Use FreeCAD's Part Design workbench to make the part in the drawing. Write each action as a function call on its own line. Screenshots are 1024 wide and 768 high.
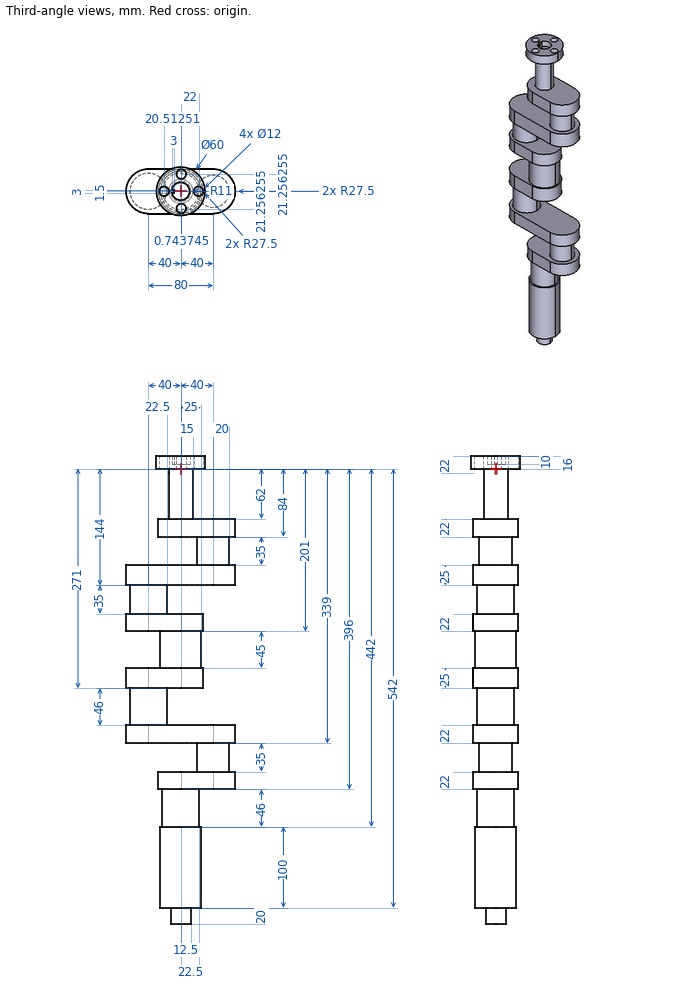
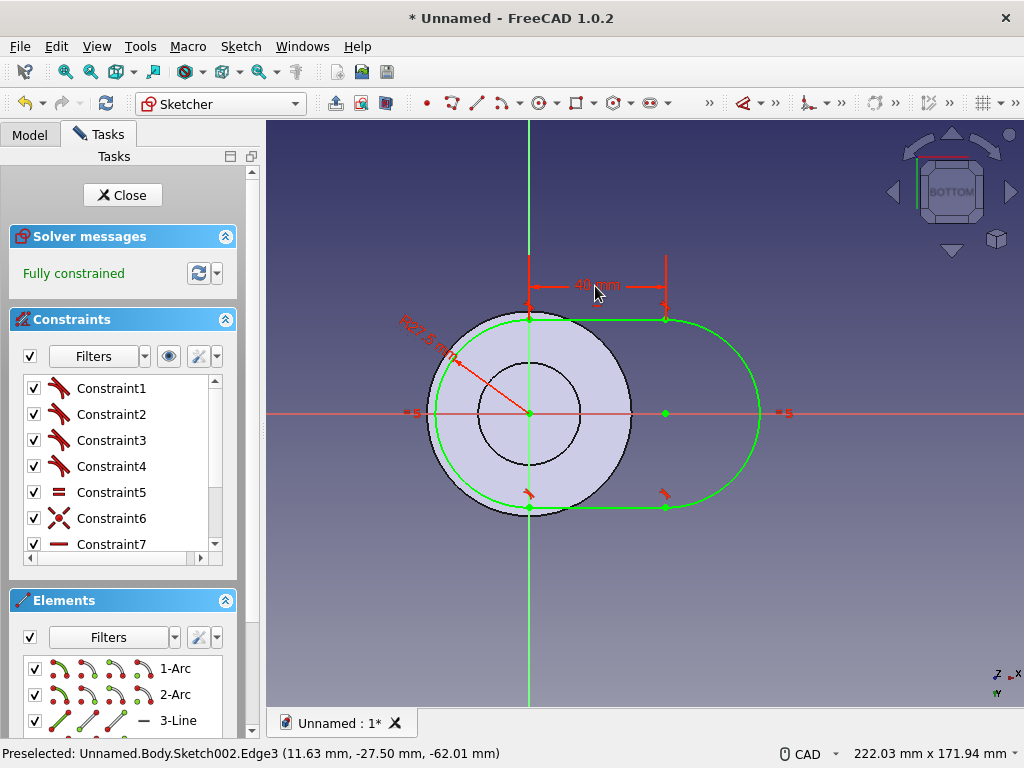
click(123, 195)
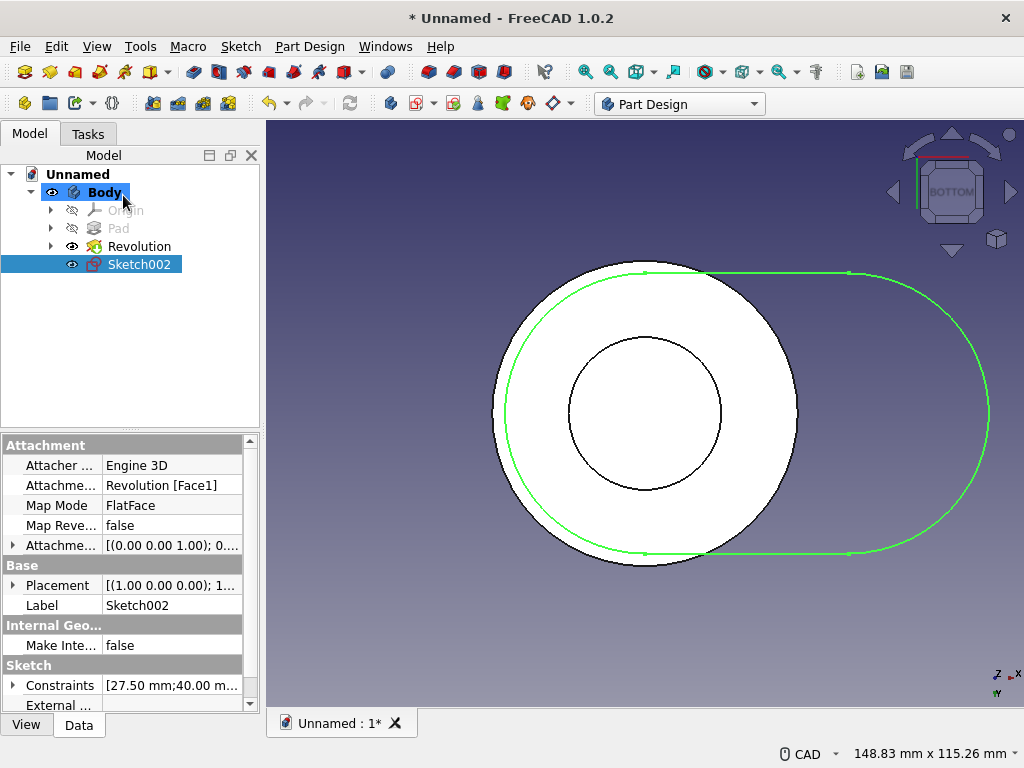
click(25, 72)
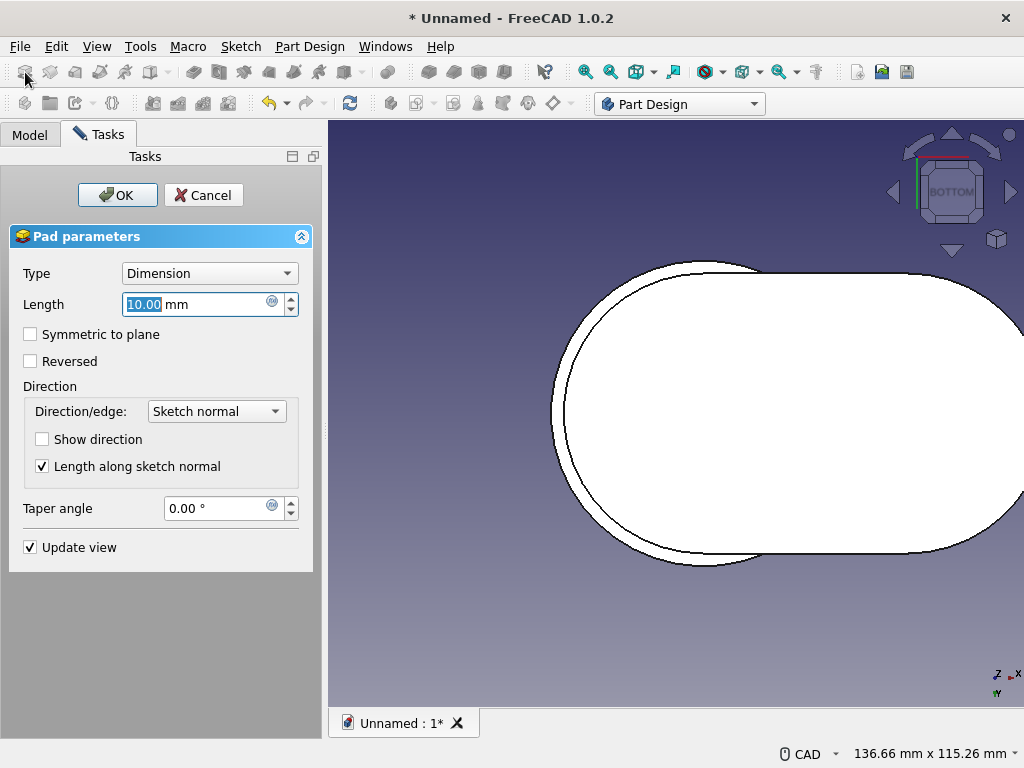
text(22)
key(Tab)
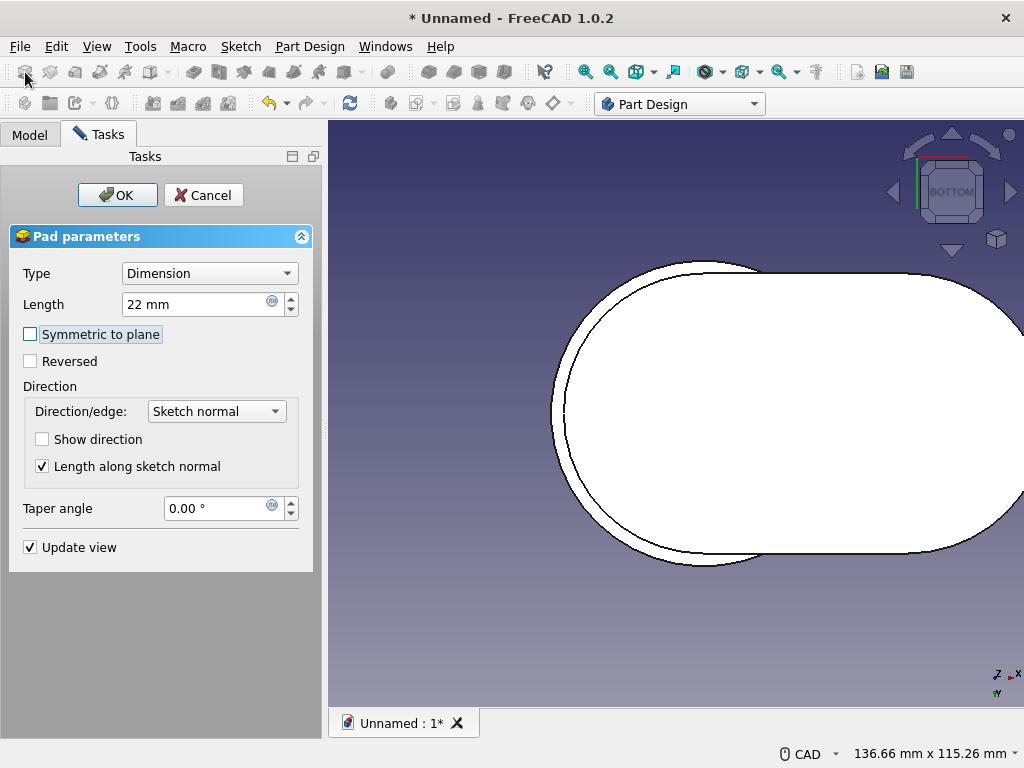
click(118, 195)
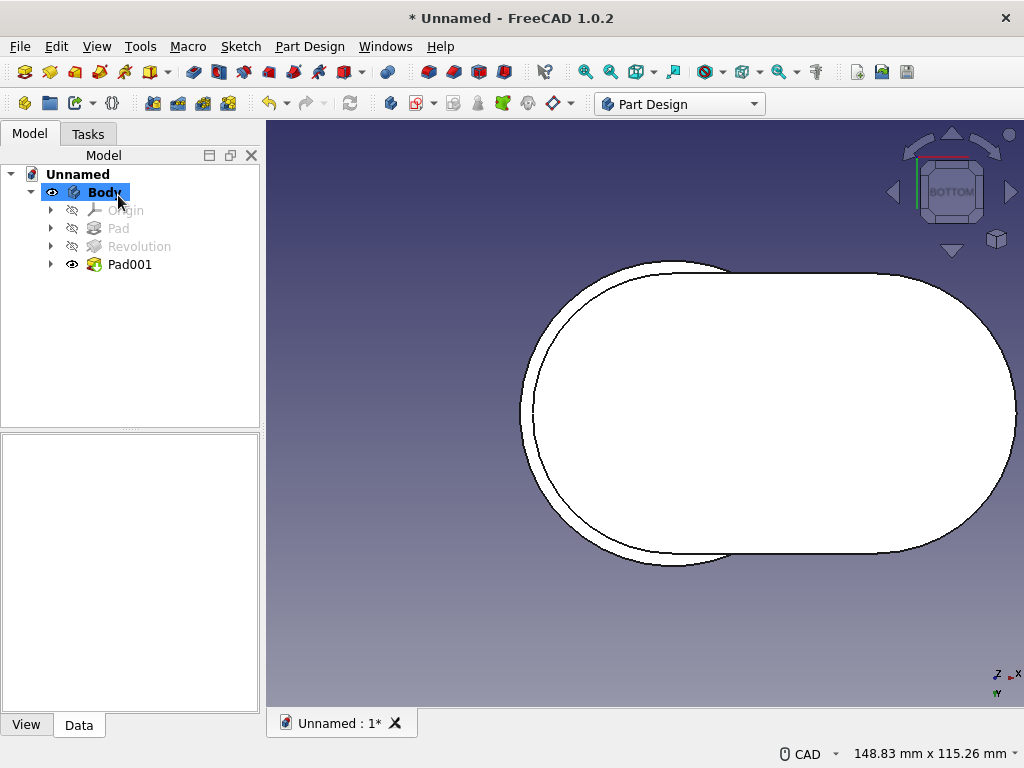
click(416, 104)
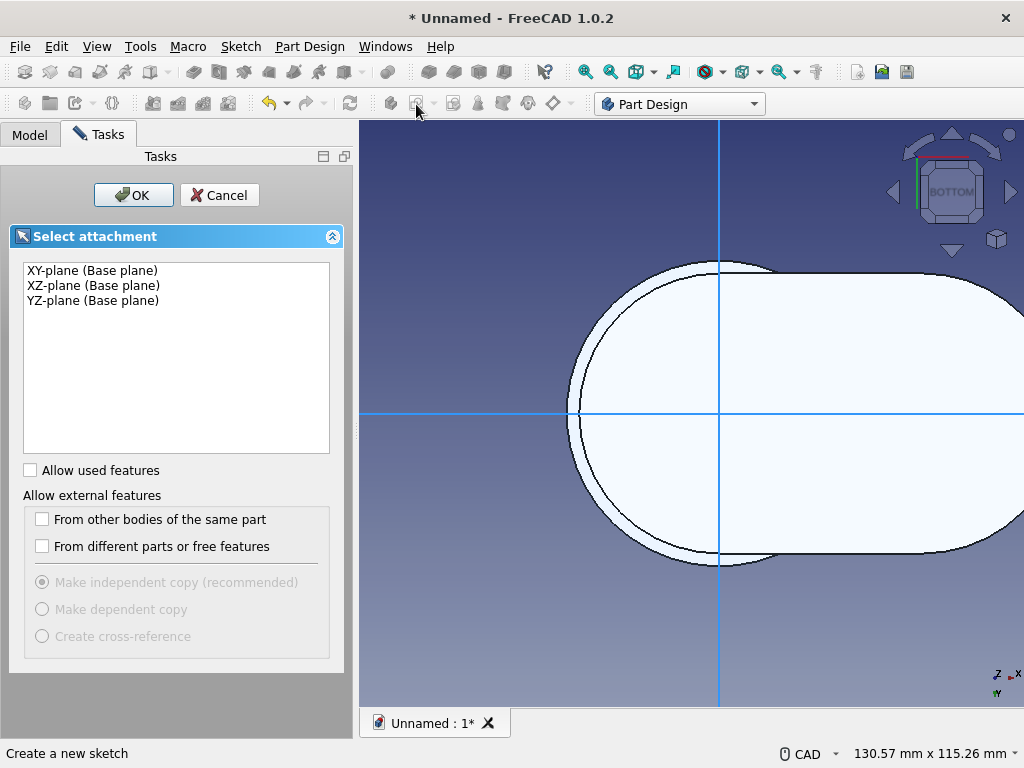
click(84, 286)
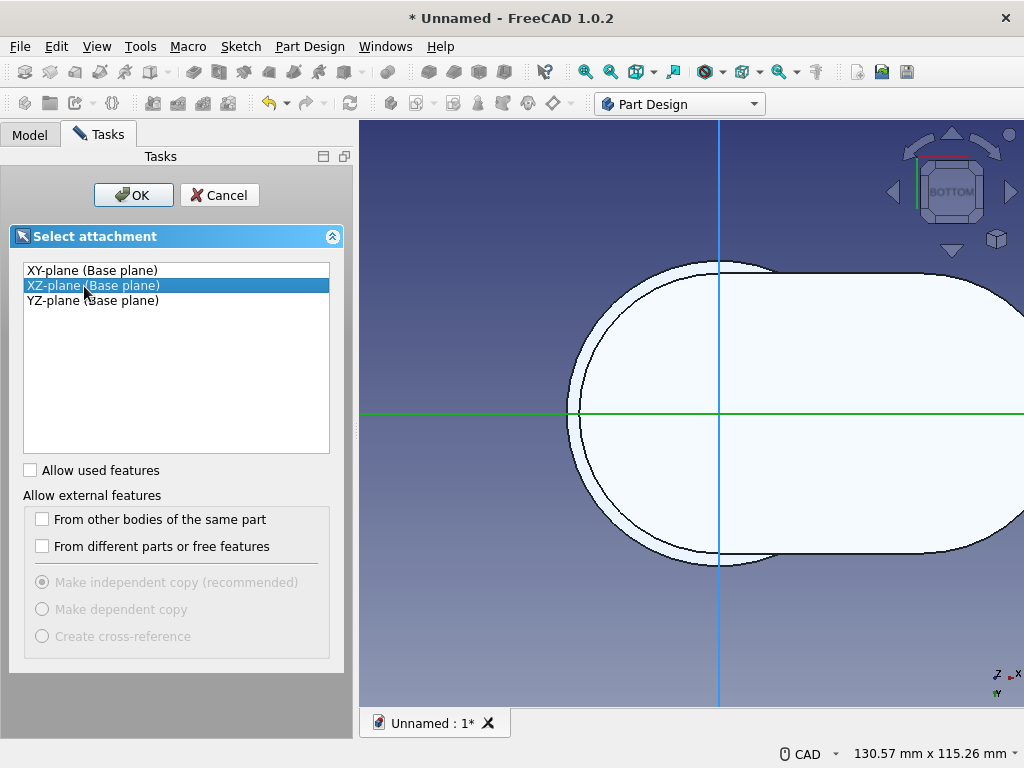
click(134, 195)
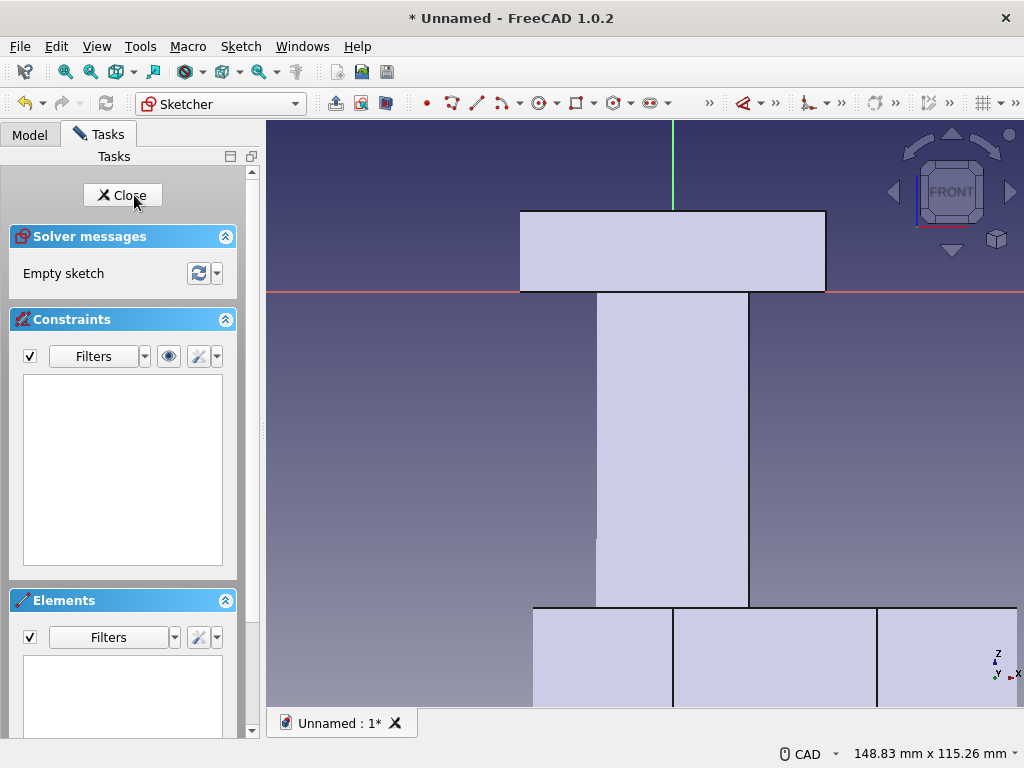
key(q)
key(s)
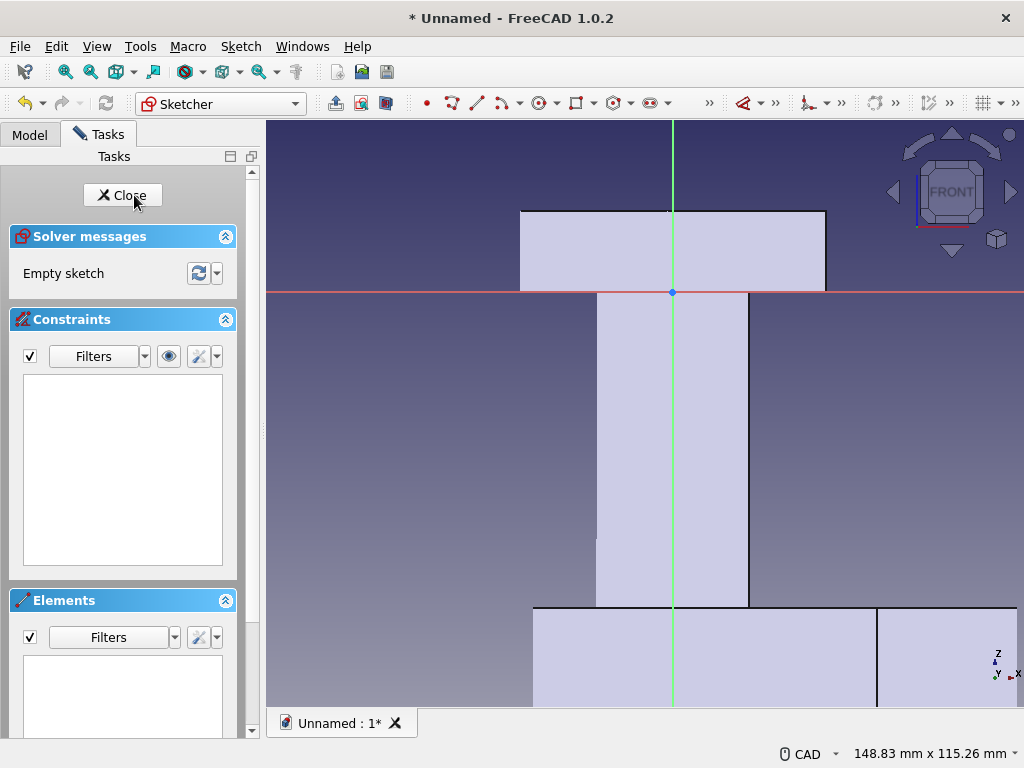
scroll(576, 414, down, 5)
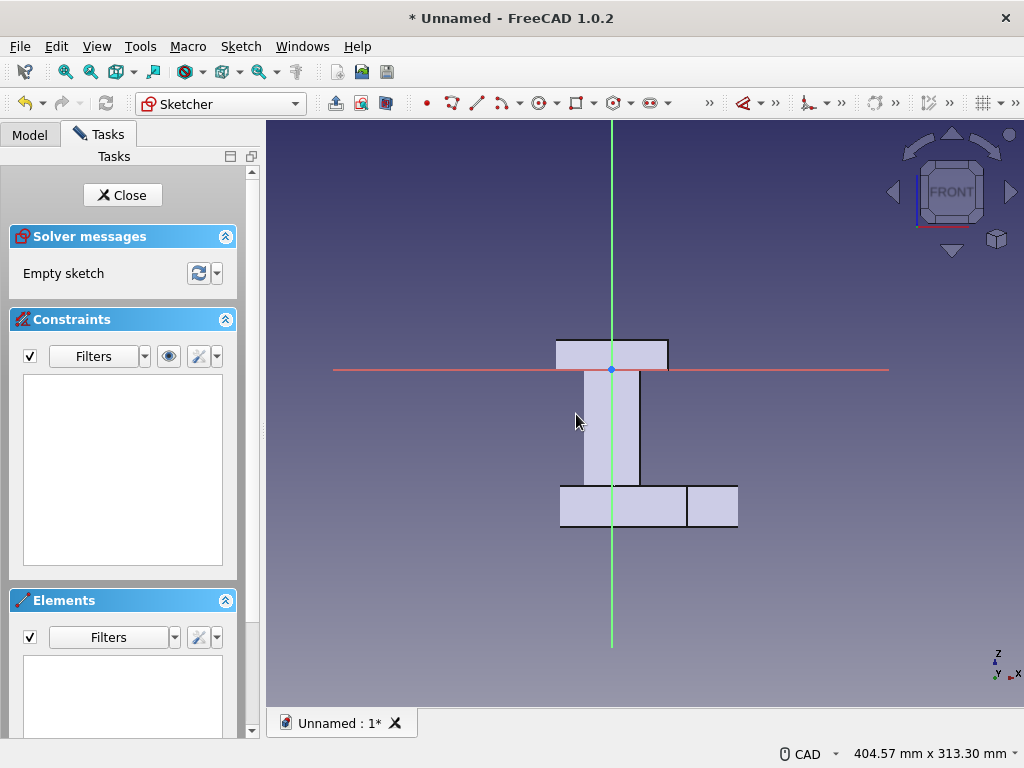
scroll(748, 625, up, 7)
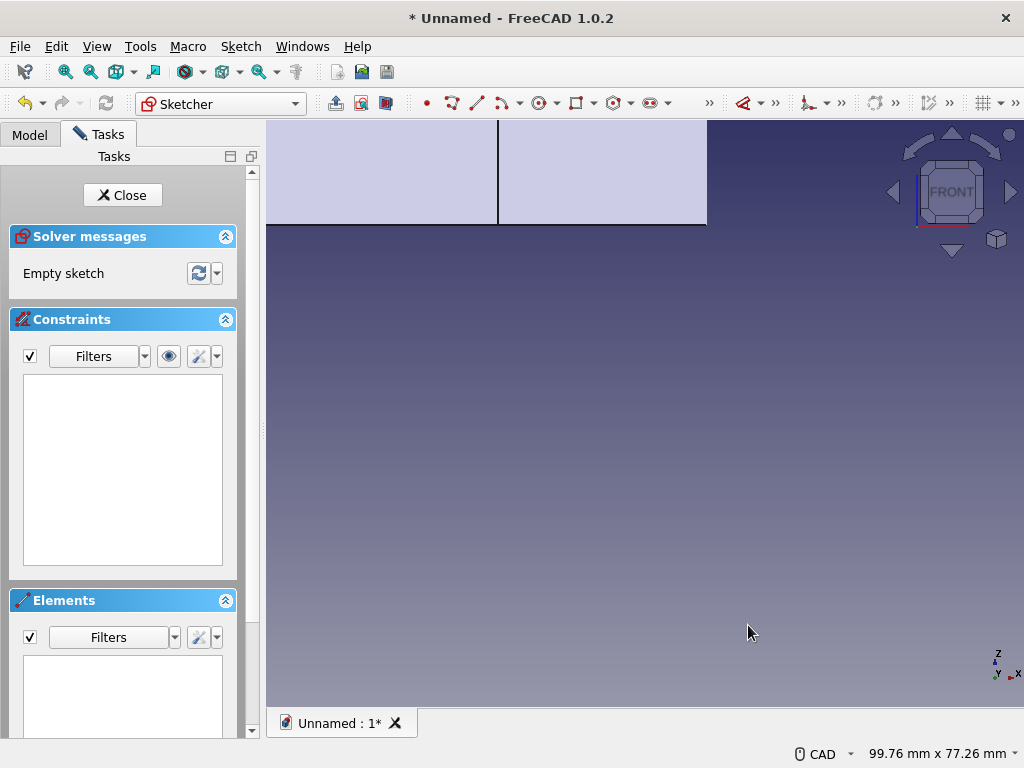
key(g)
key(r)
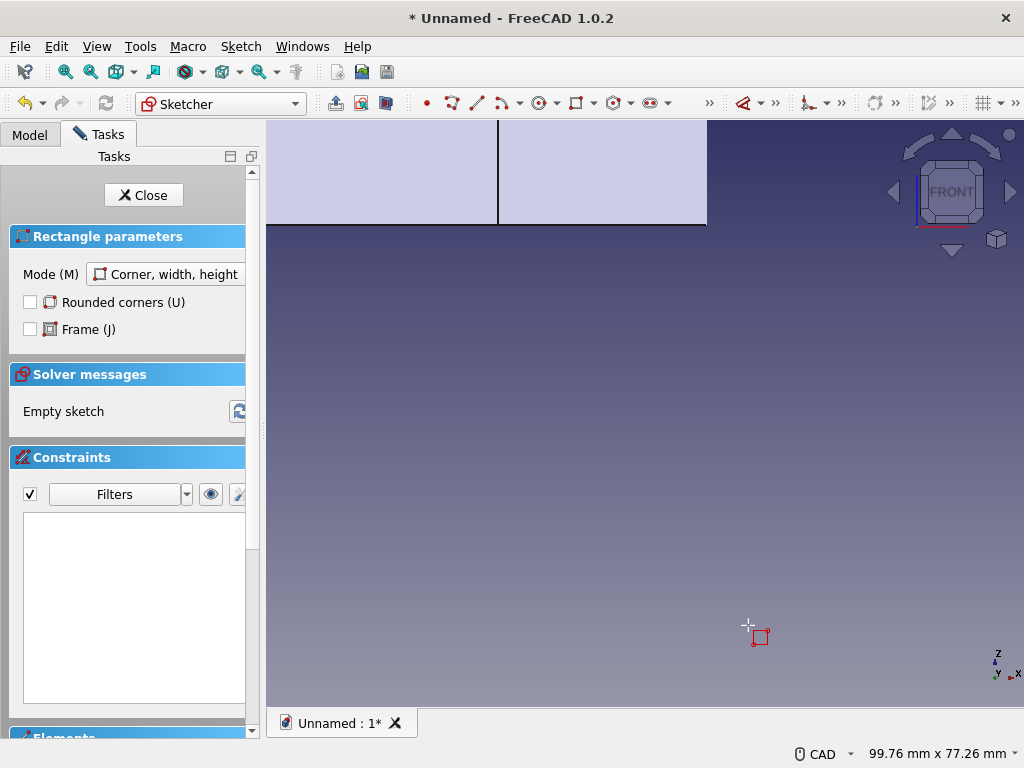
click(498, 225)
move(650, 490)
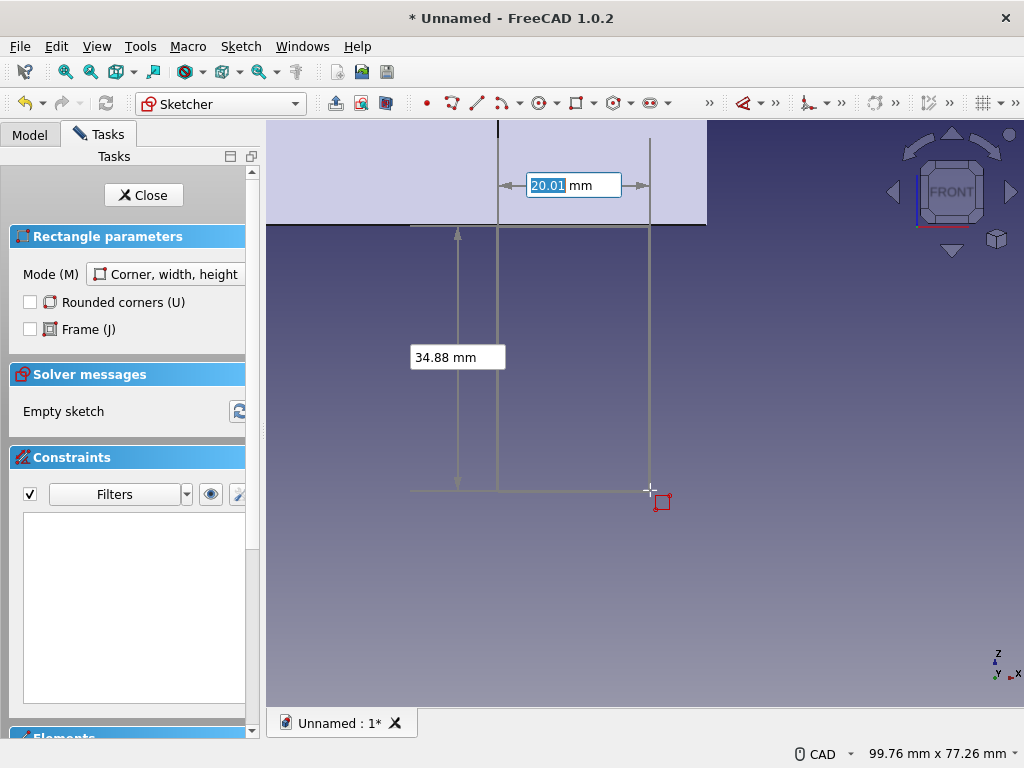
text(20)
key(Tab)
text(35)
key(Return)